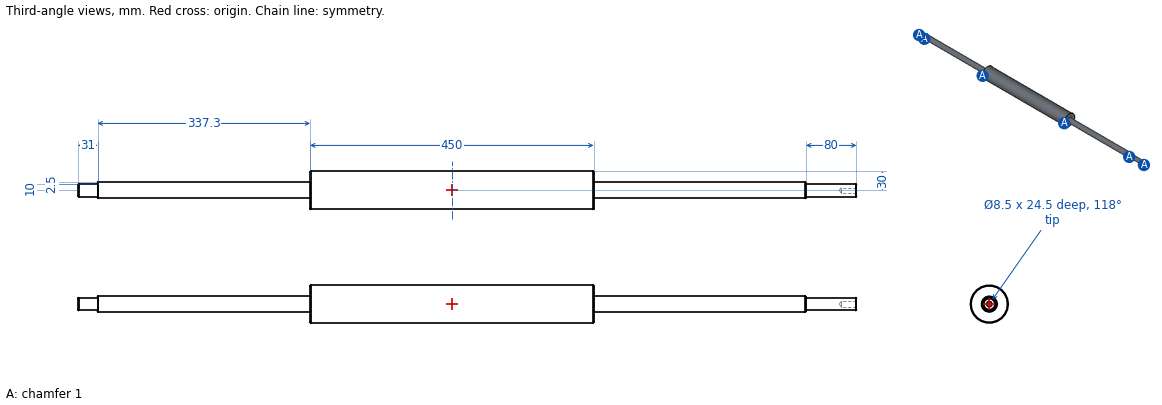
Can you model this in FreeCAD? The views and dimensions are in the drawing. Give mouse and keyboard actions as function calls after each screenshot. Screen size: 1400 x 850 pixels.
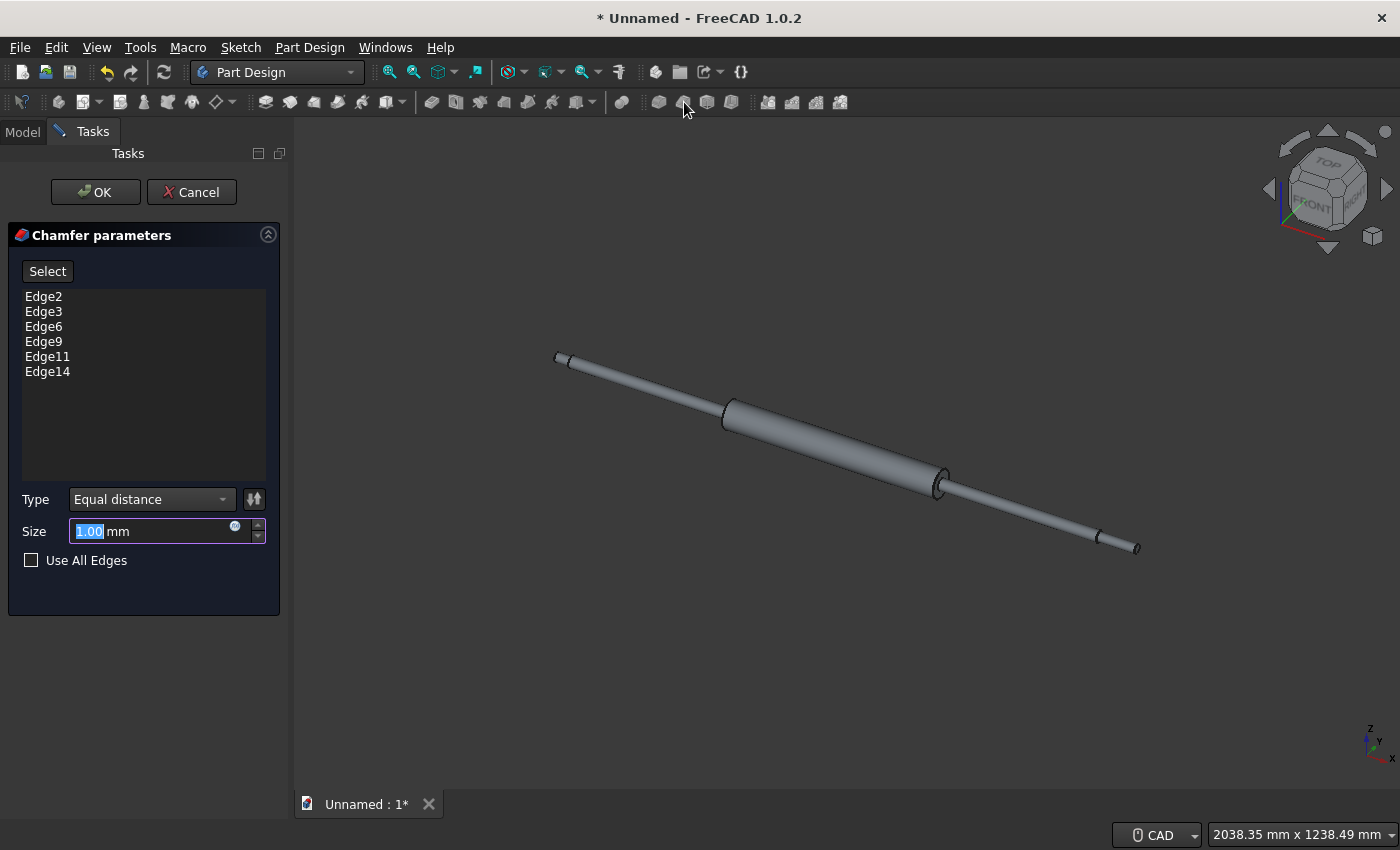
text(1)
key(Tab)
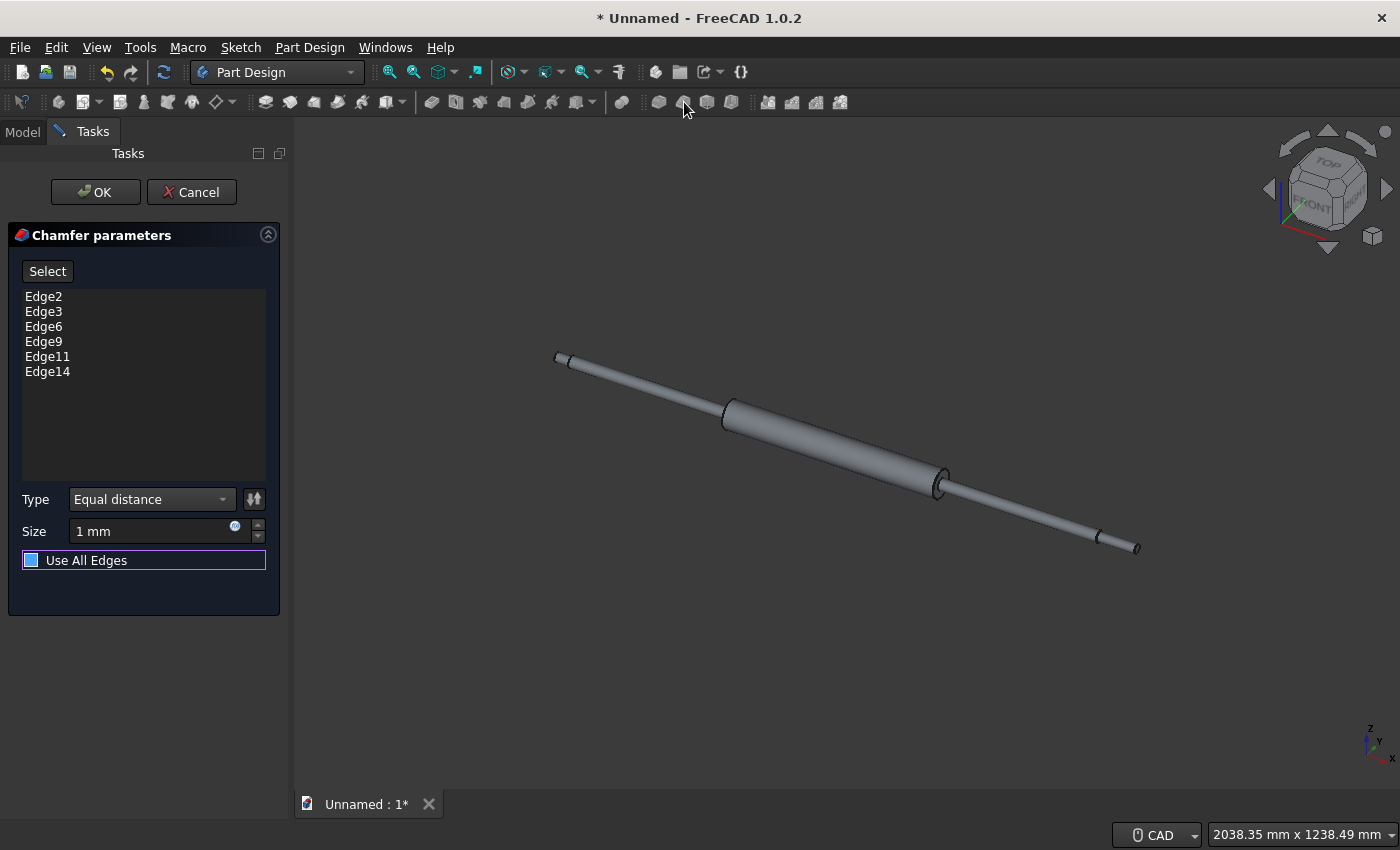
click(96, 192)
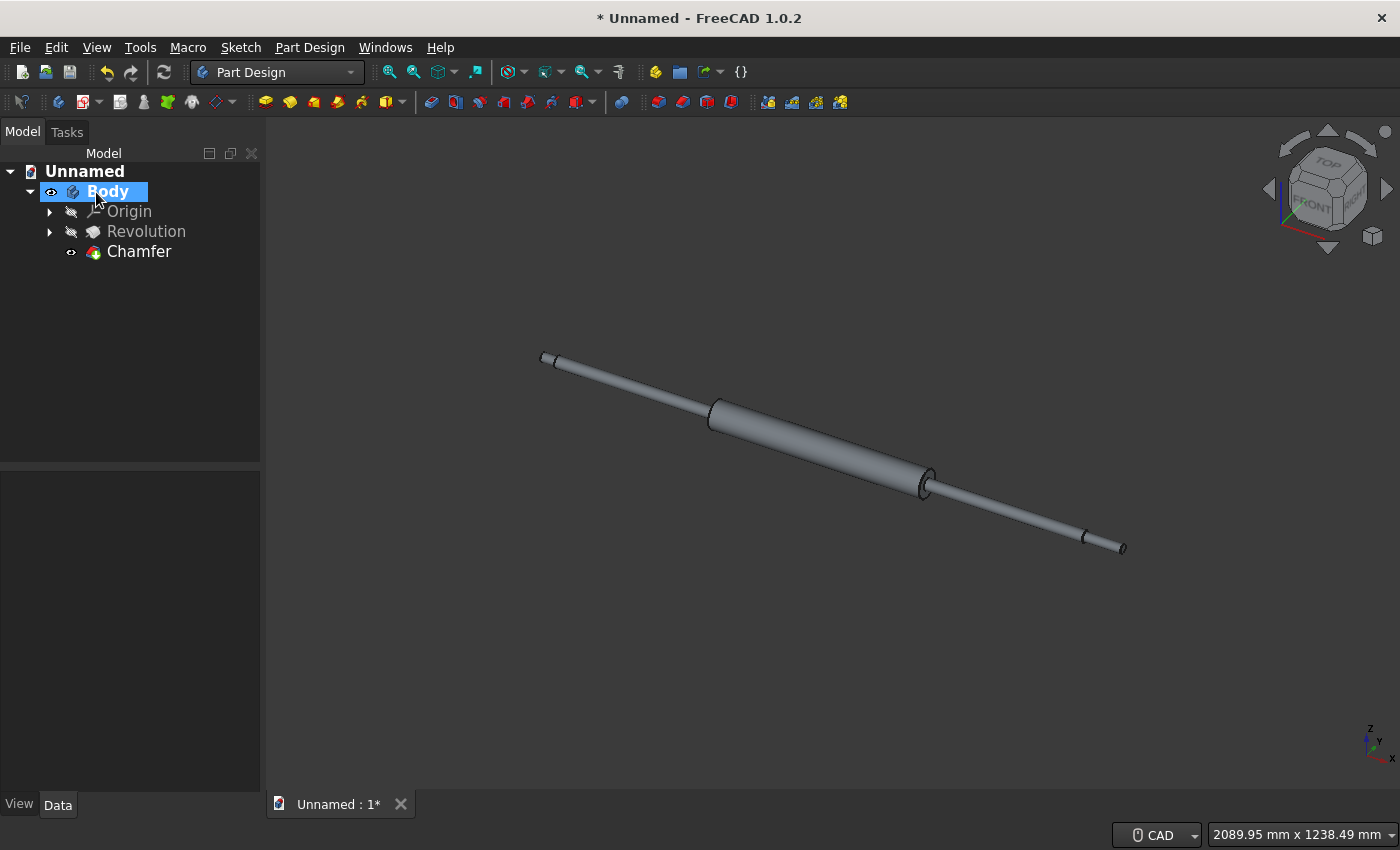
scroll(1123, 548, up, 5)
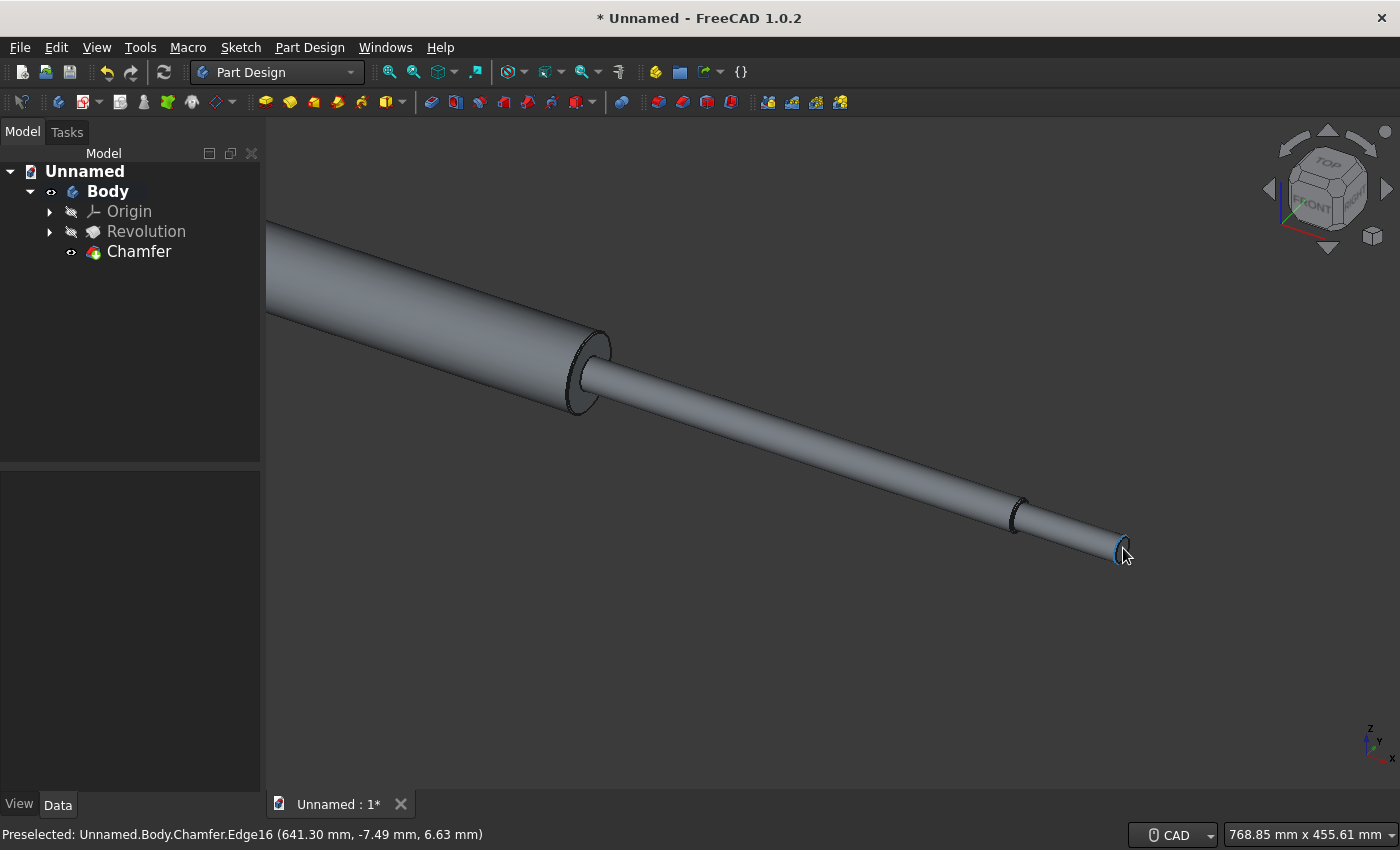
click(390, 72)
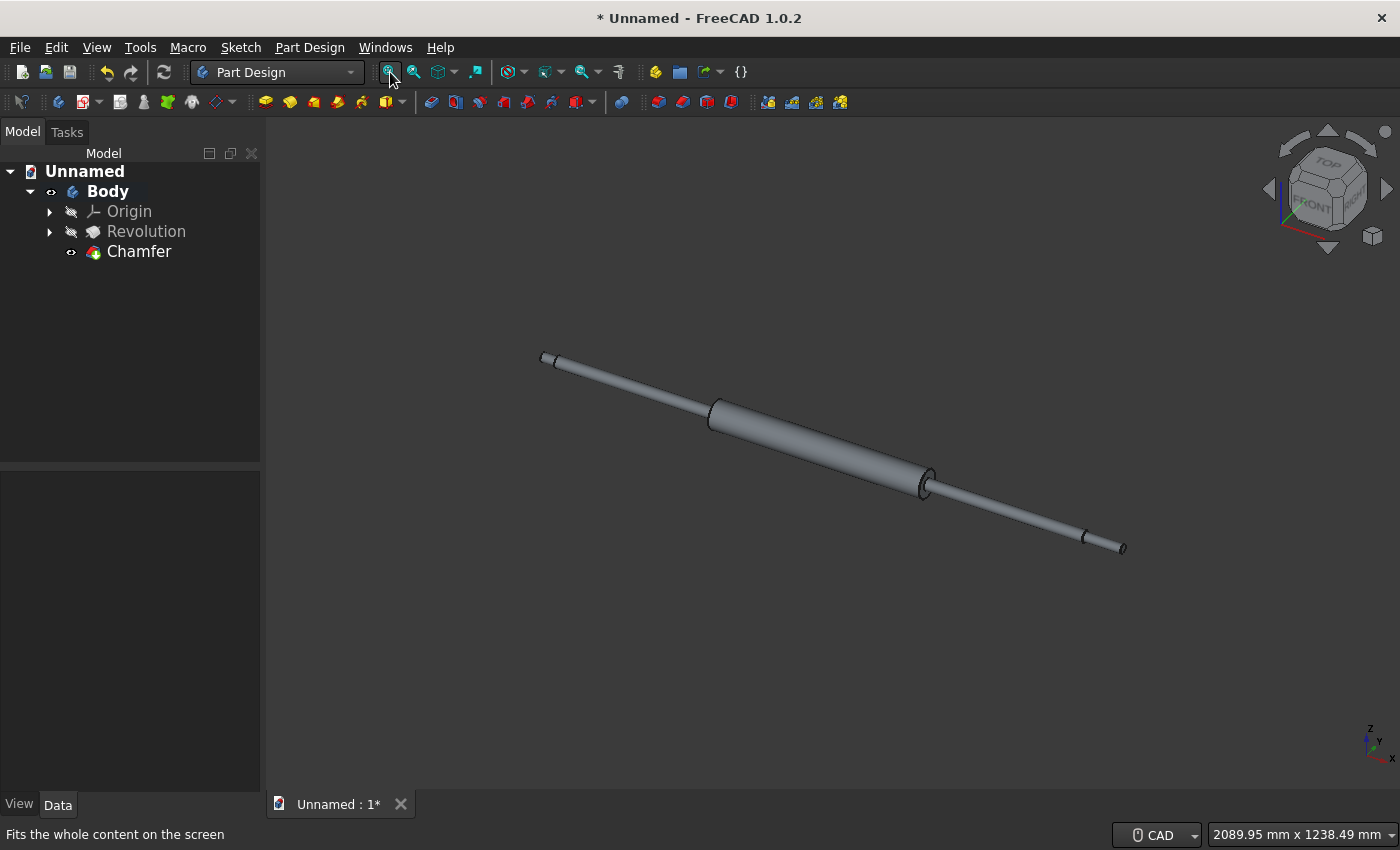
key(0)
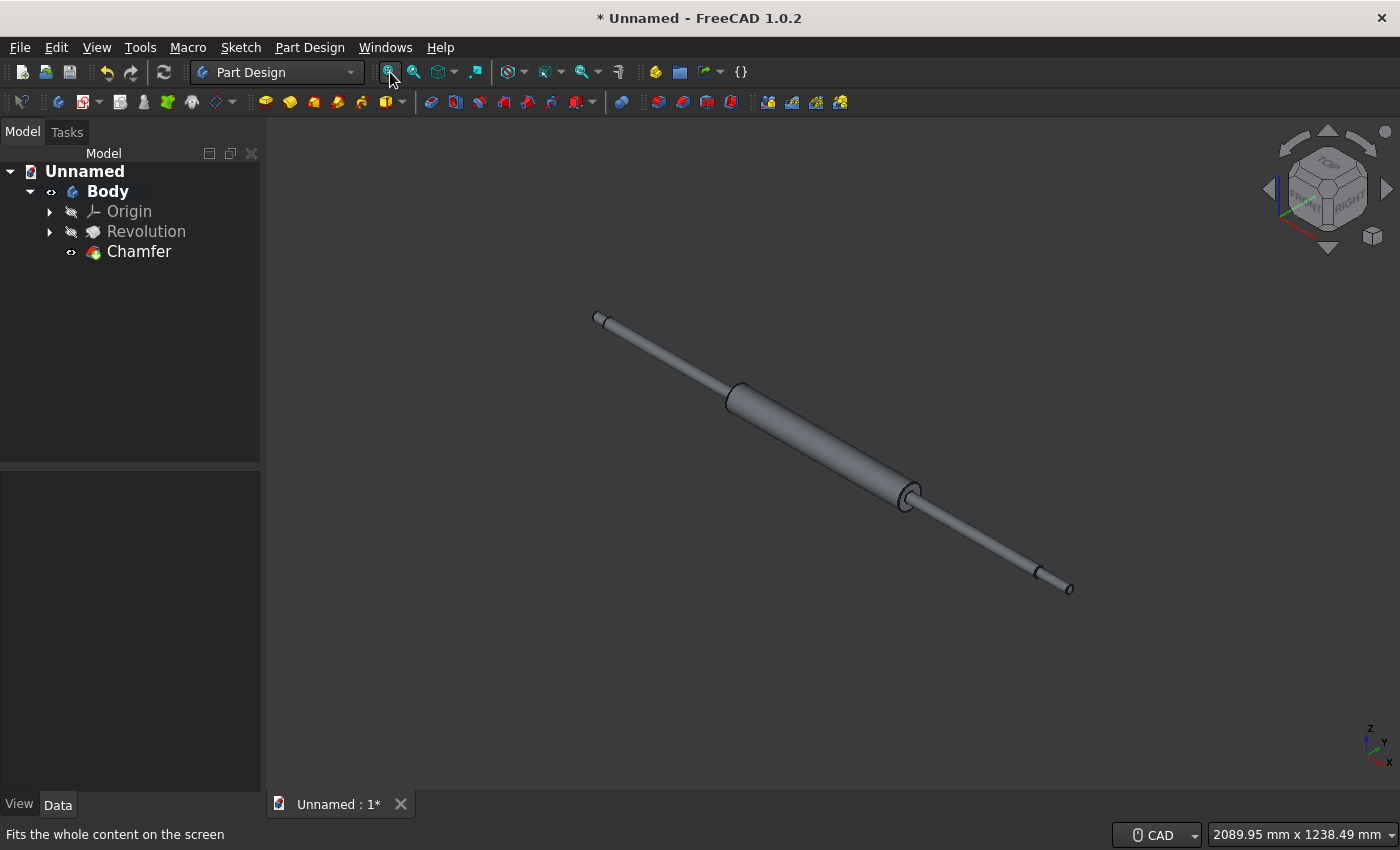
scroll(1070, 589, up, 5)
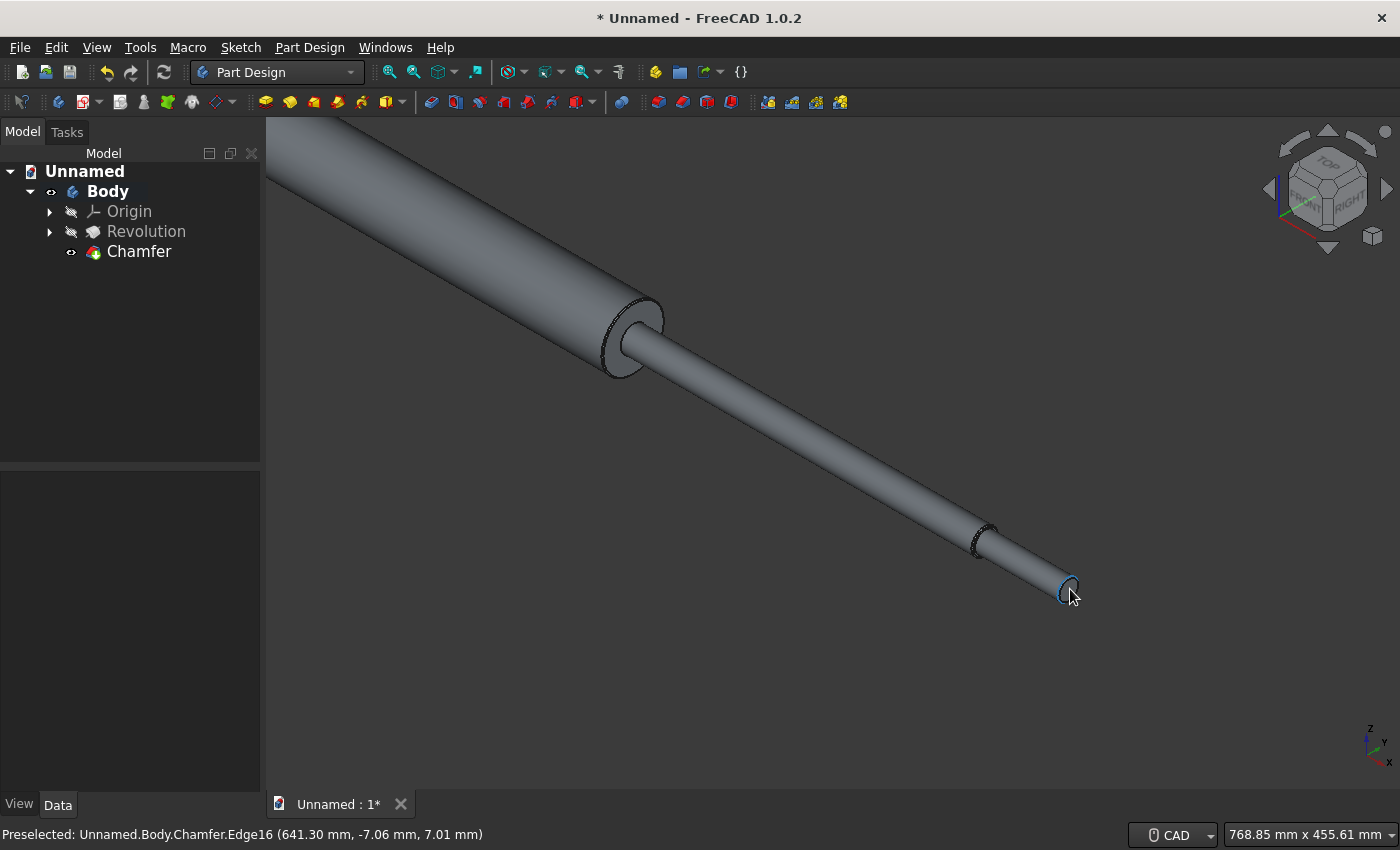
click(1072, 588)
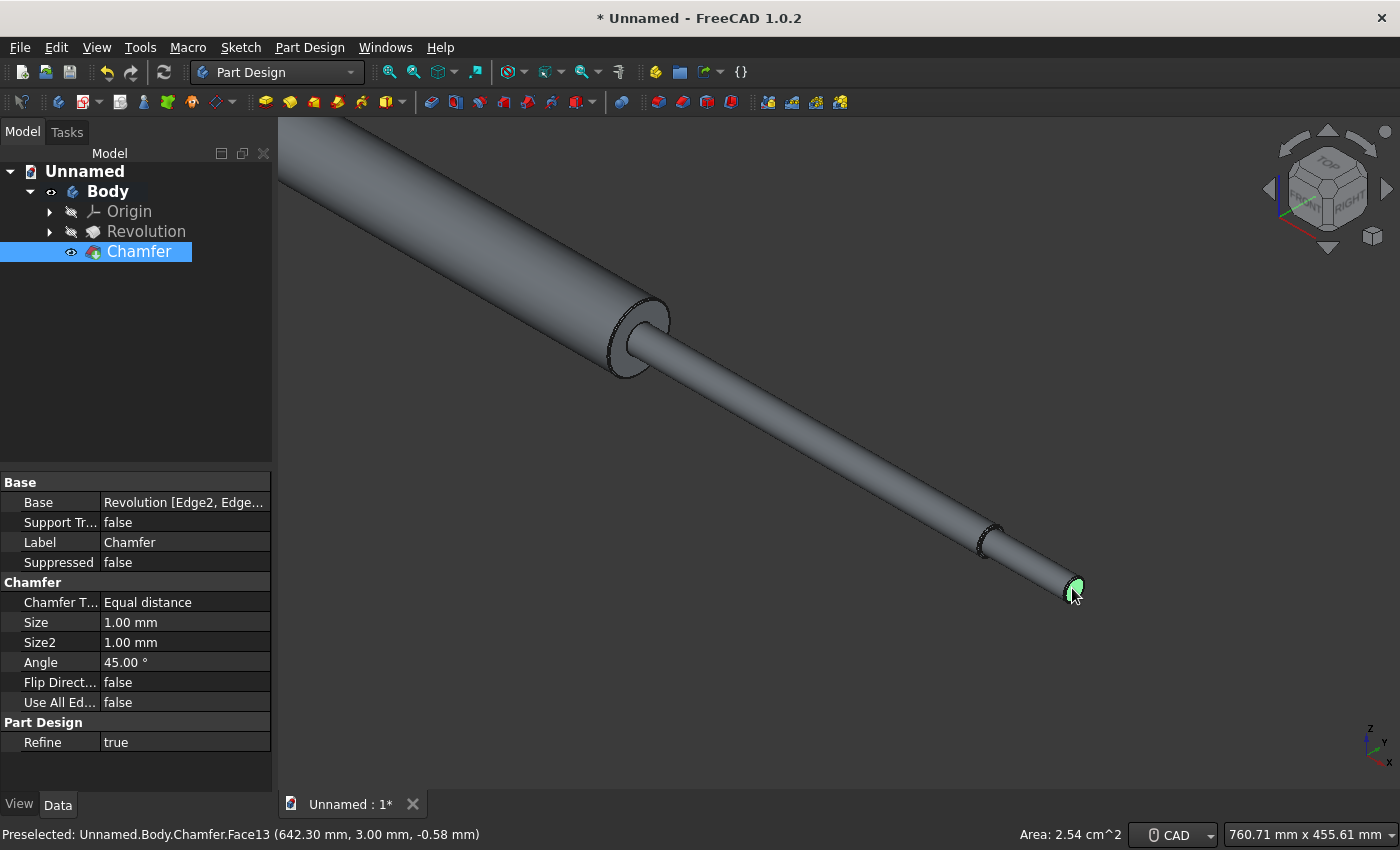
click(84, 102)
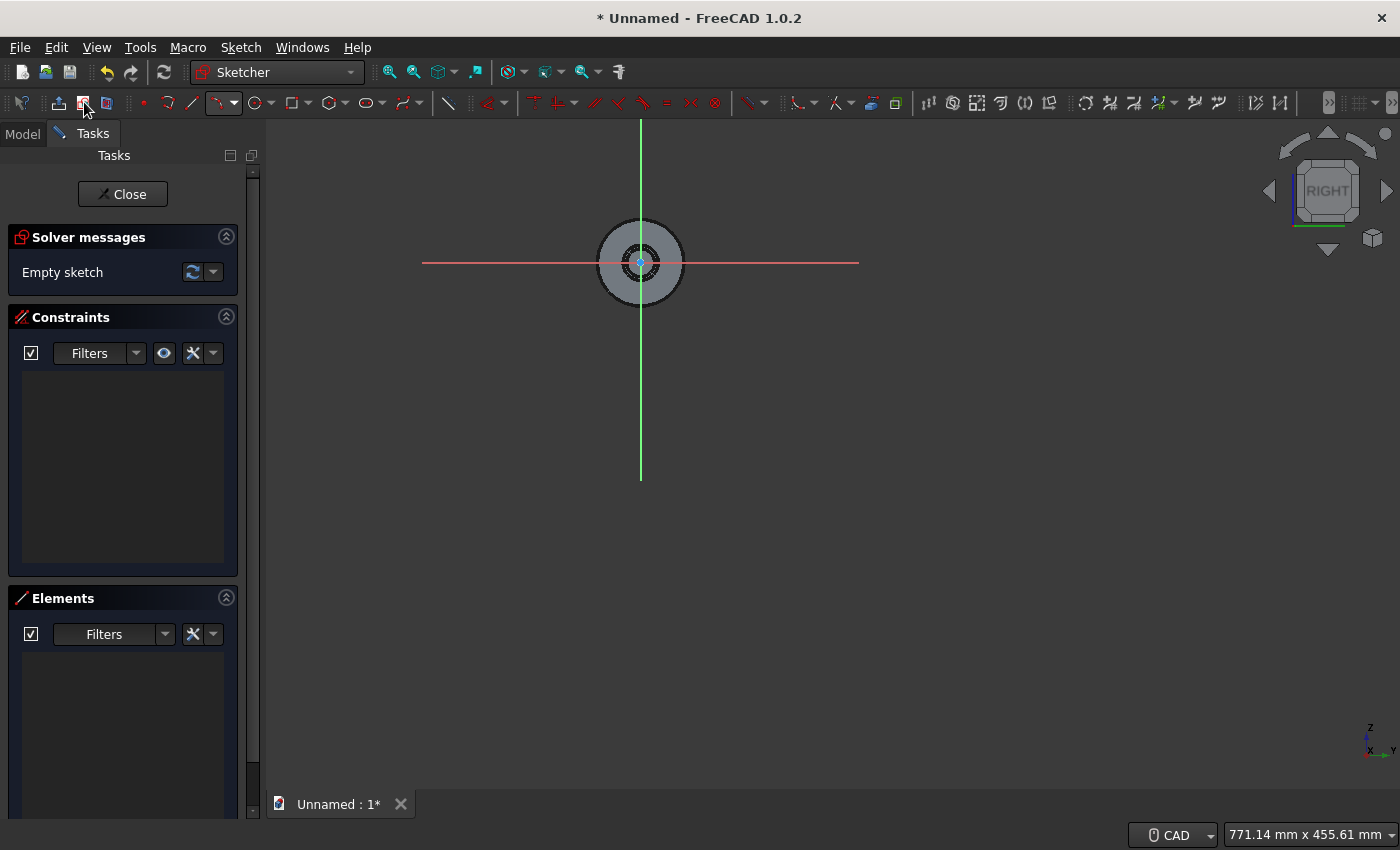
scroll(634, 253, up, 15)